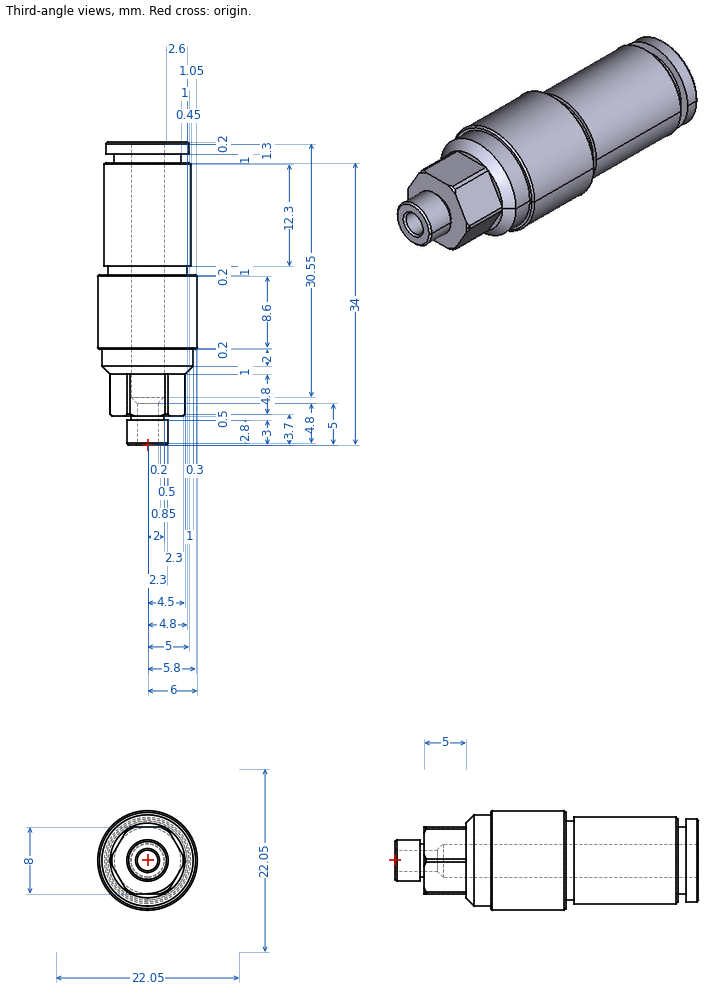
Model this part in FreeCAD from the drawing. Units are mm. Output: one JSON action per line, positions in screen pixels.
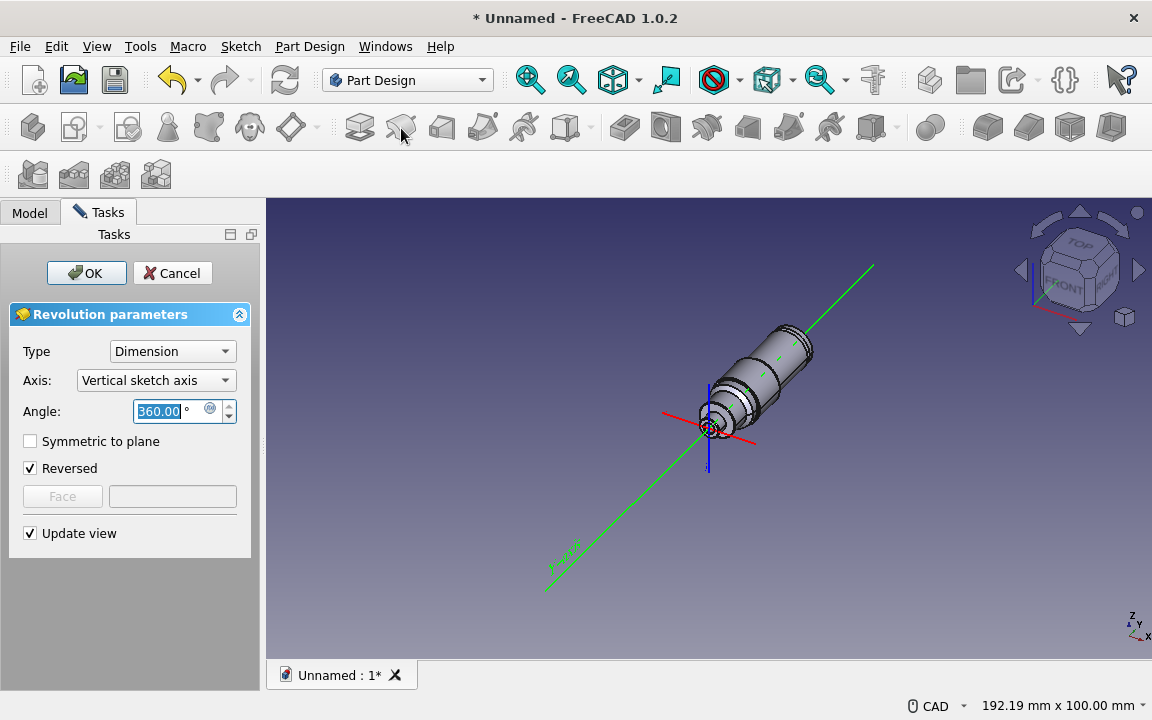
{"action": "left_click", "coordinate": [87, 273]}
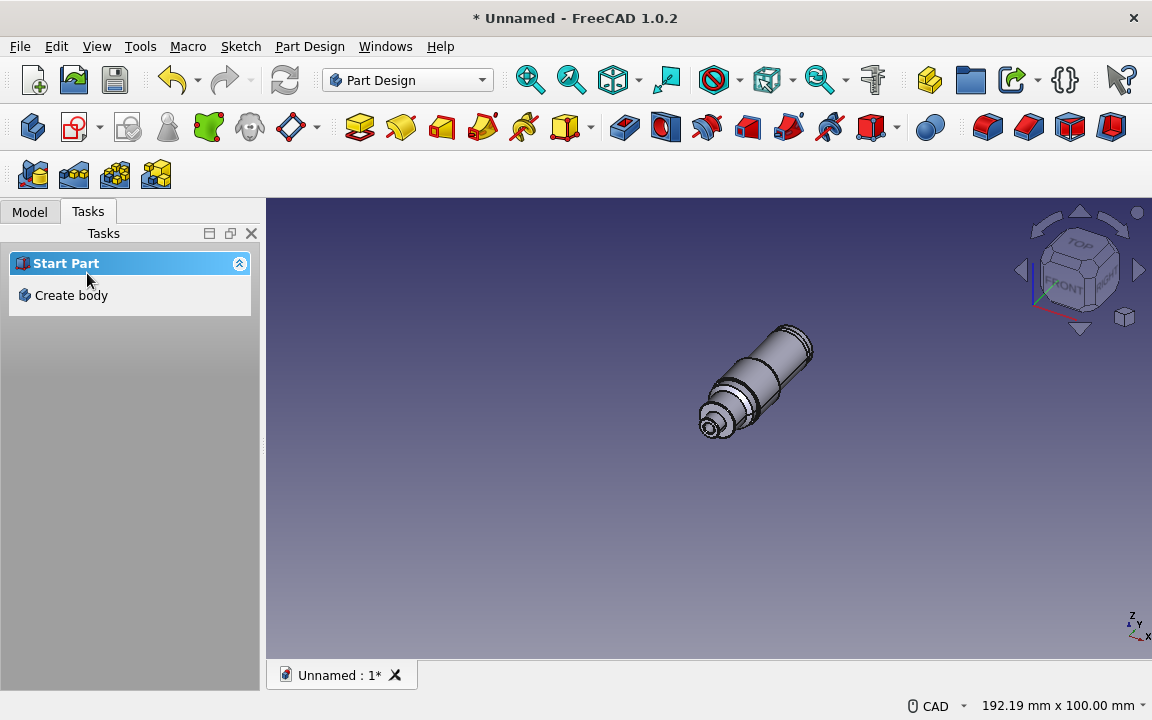
{"action": "left_click", "coordinate": [531, 80]}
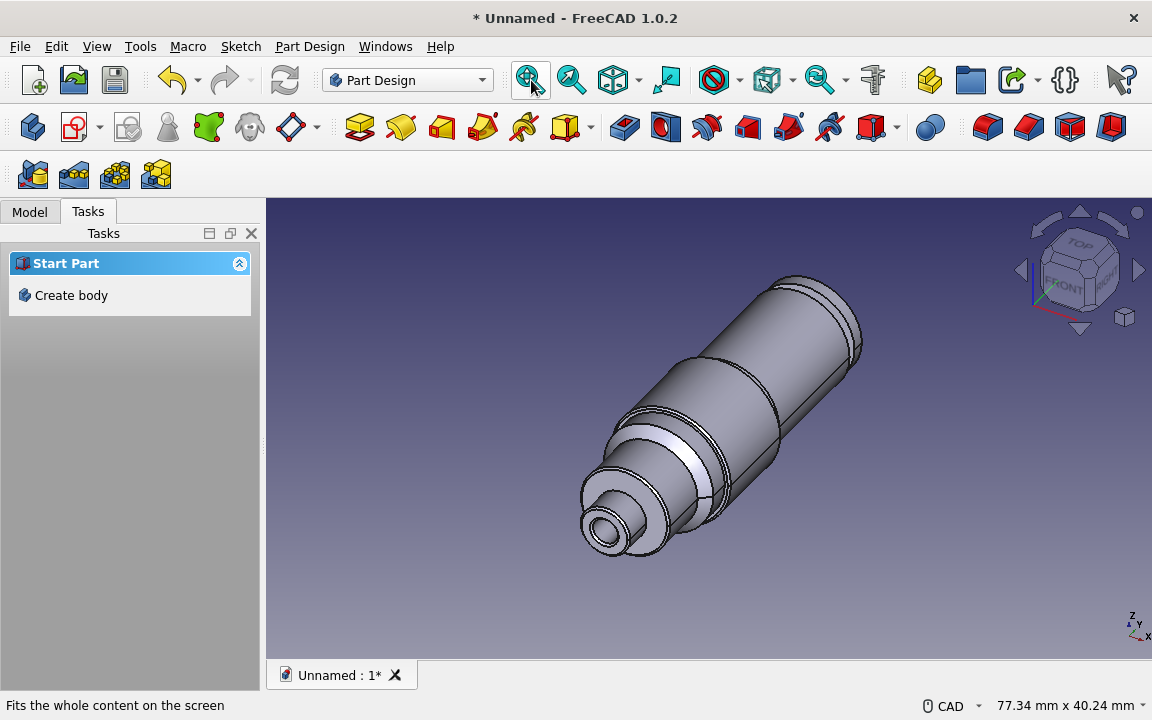
{"action": "left_click", "coordinate": [649, 543]}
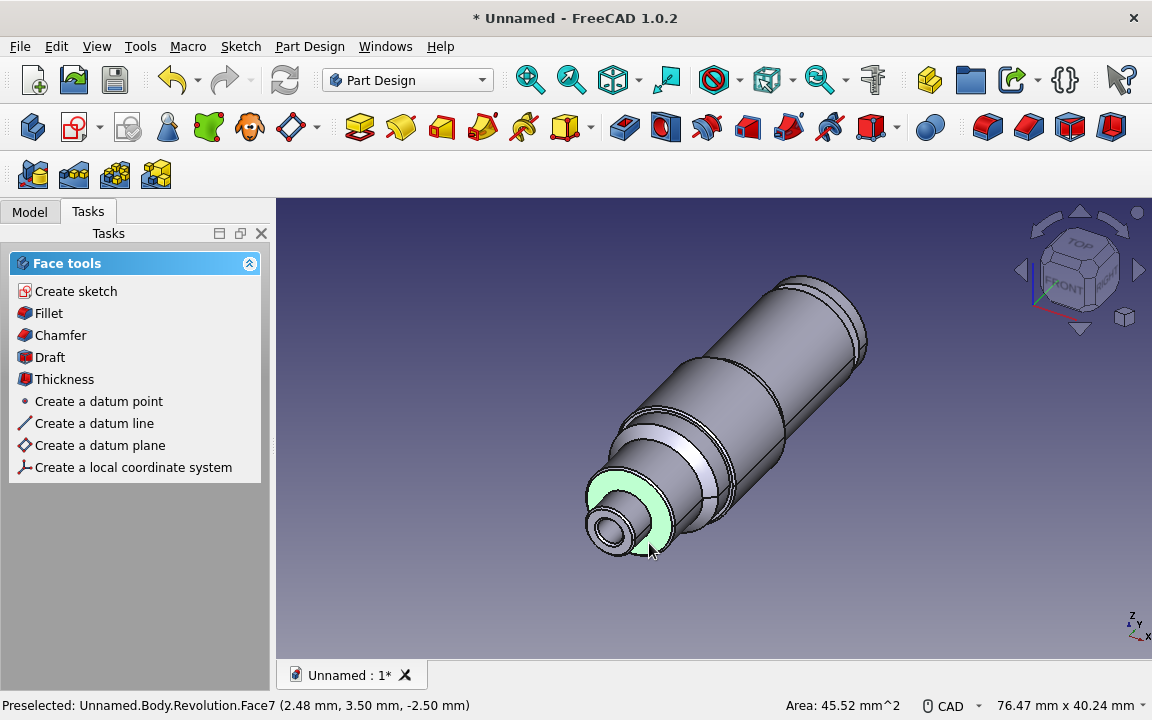
{"action": "left_click", "coordinate": [74, 128]}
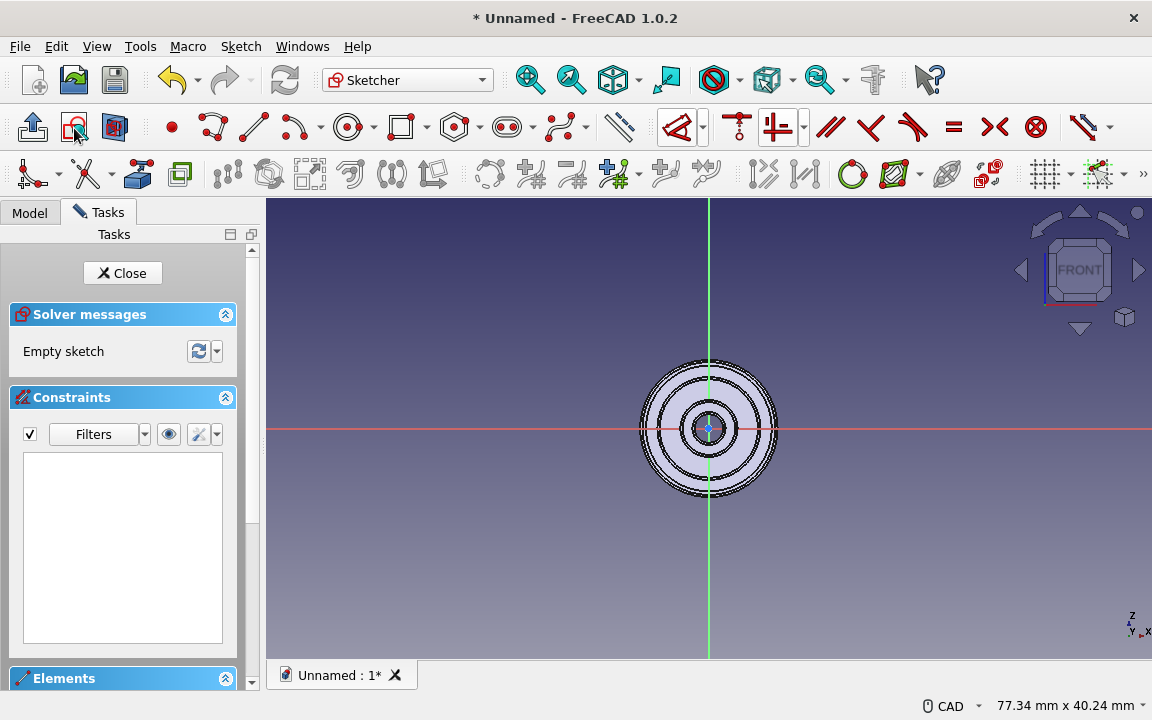
{"action": "left_click", "coordinate": [426, 128]}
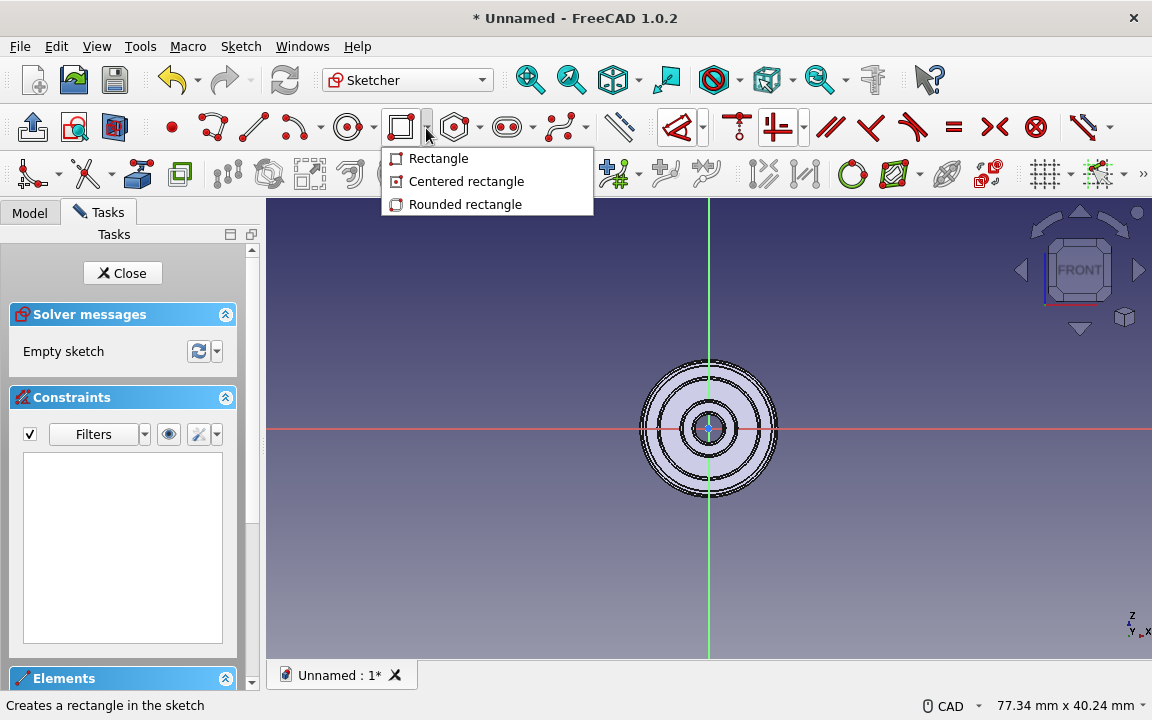
{"action": "left_click", "coordinate": [488, 182]}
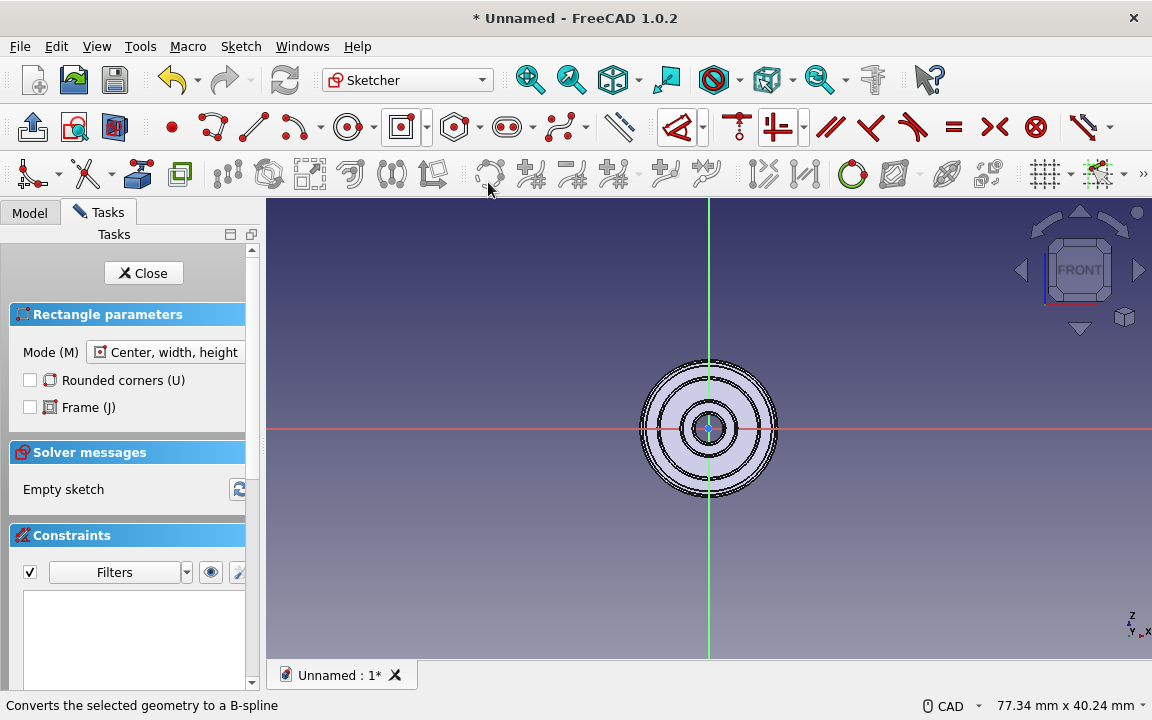
{"action": "left_click", "coordinate": [709, 429]}
{"action": "mouse_move", "coordinate": [835, 302]}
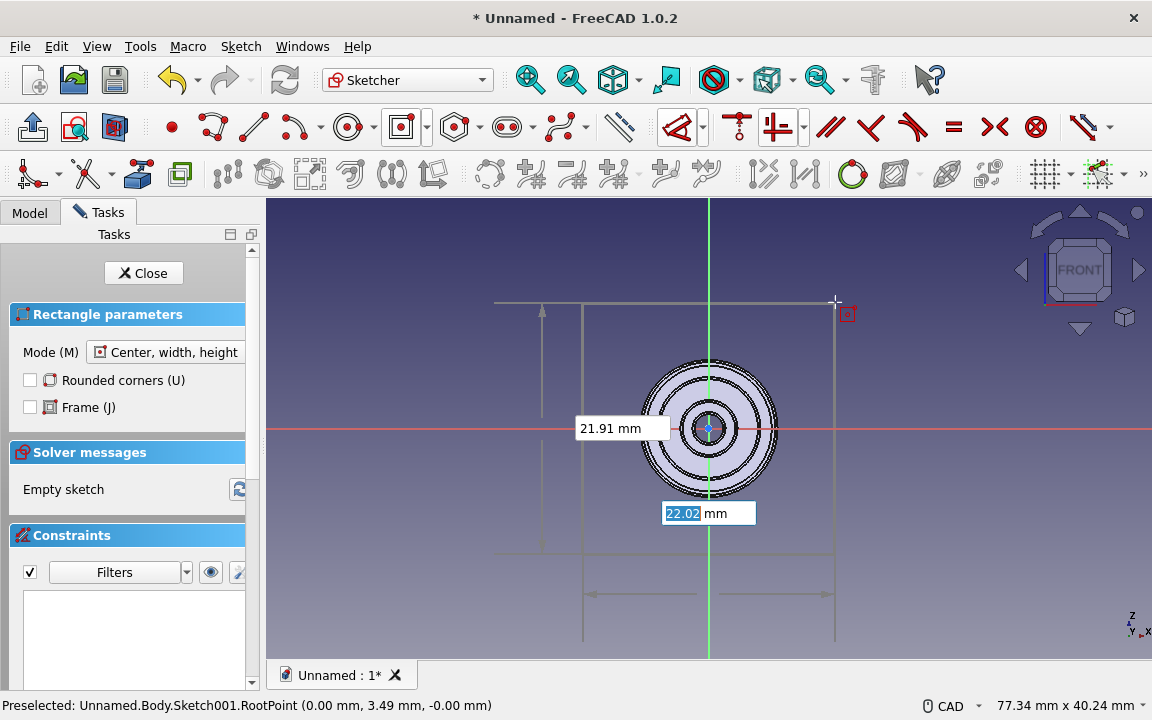
{"action": "type", "text": "22.05"}
{"action": "key", "text": "Tab"}
{"action": "type", "text": "22.05"}
{"action": "key", "text": "Return"}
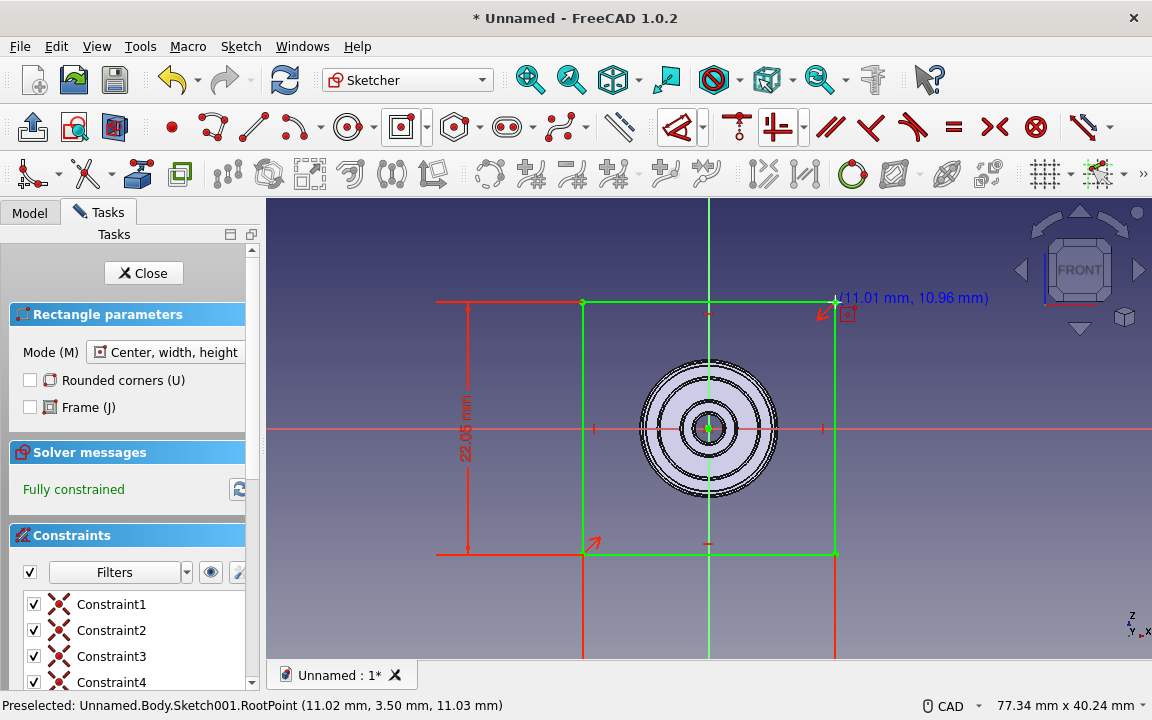
{"action": "left_click", "coordinate": [454, 128]}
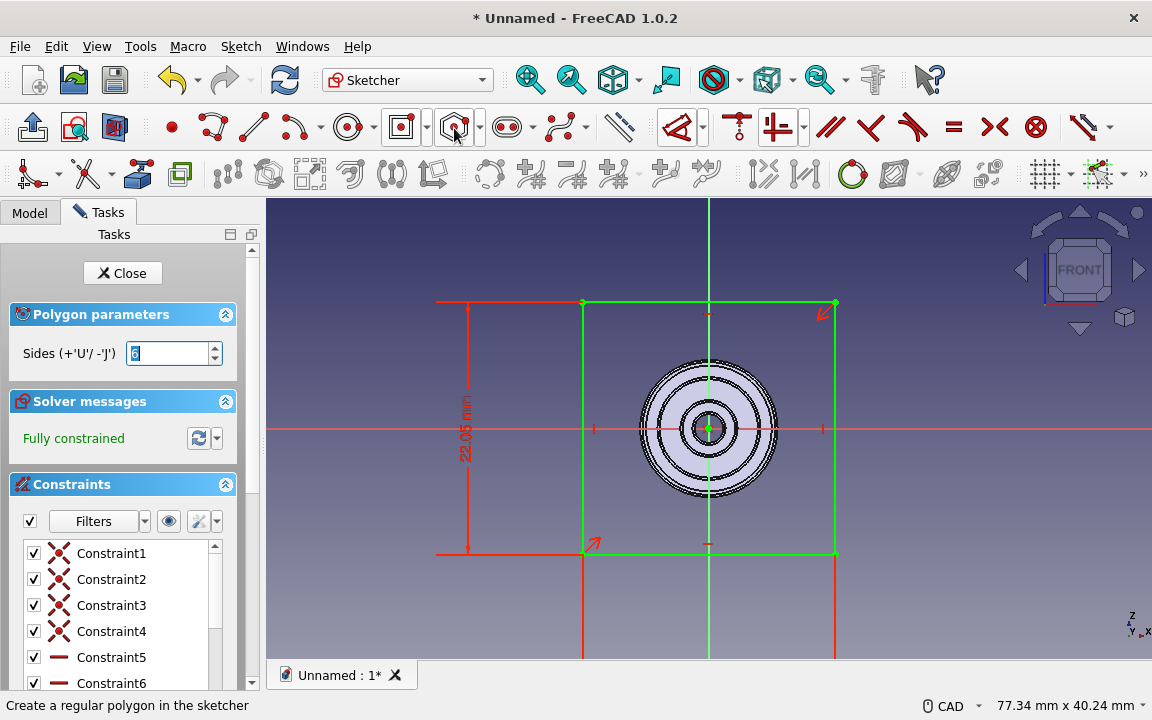
{"action": "left_click", "coordinate": [709, 429]}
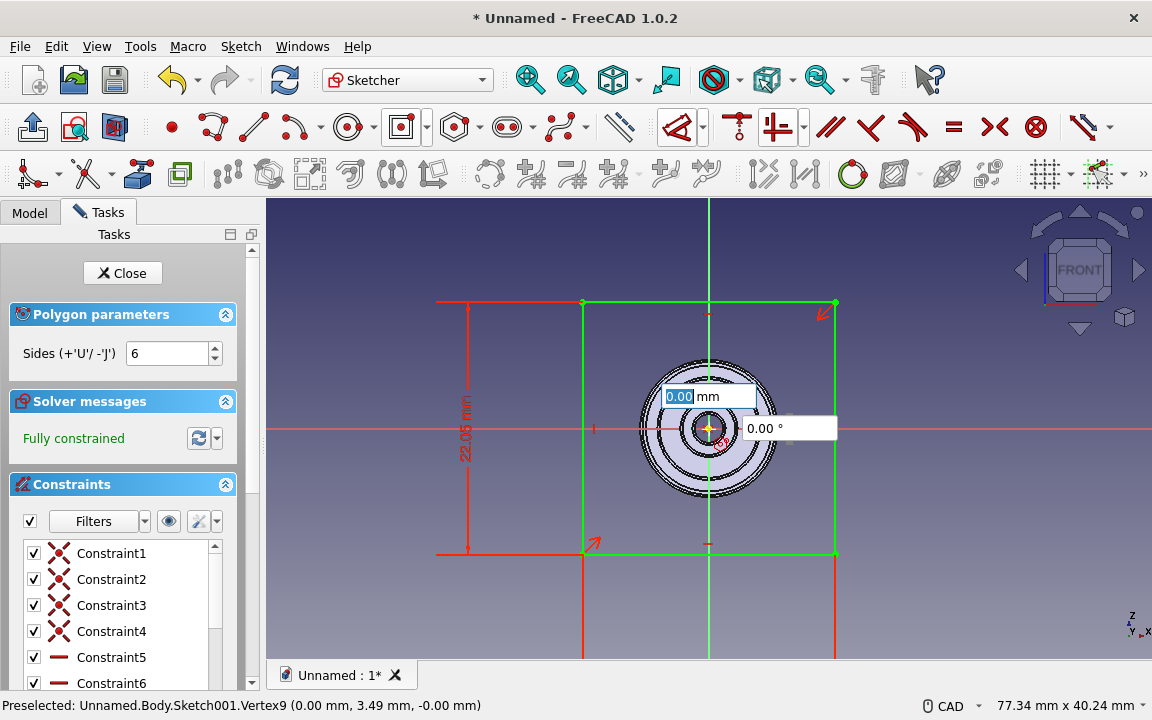
{"action": "left_click", "coordinate": [762, 429]}
{"action": "key", "text": "Escape"}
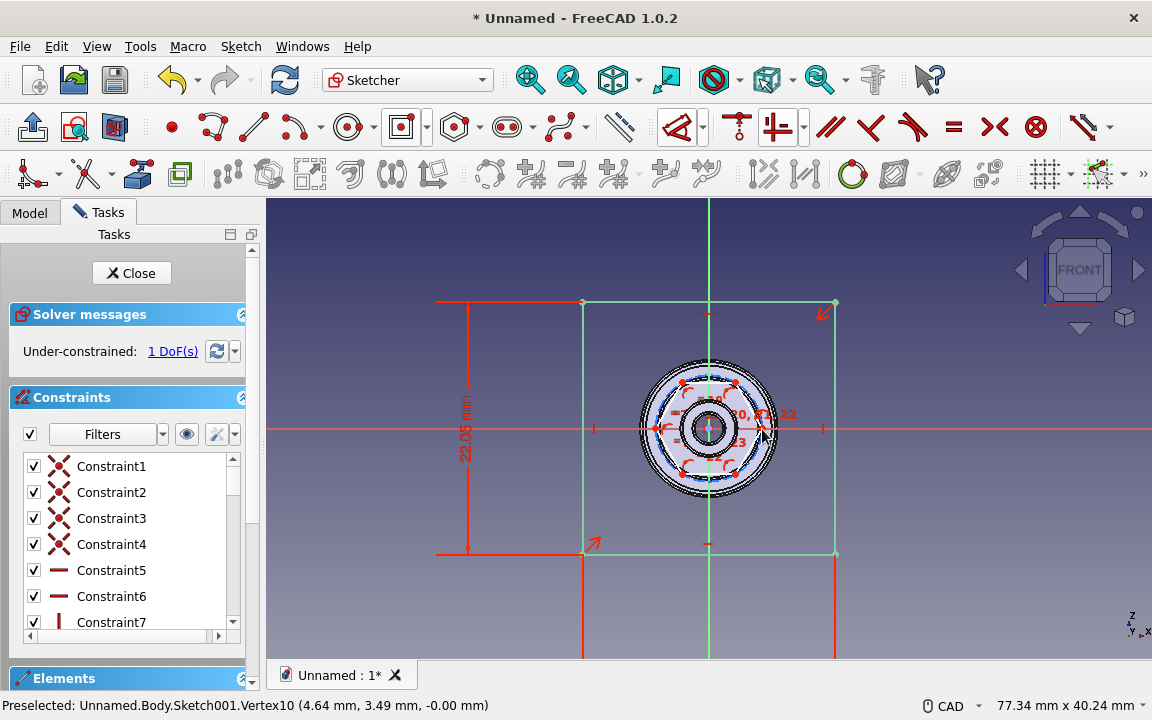
{"action": "left_click", "coordinate": [682, 474]}